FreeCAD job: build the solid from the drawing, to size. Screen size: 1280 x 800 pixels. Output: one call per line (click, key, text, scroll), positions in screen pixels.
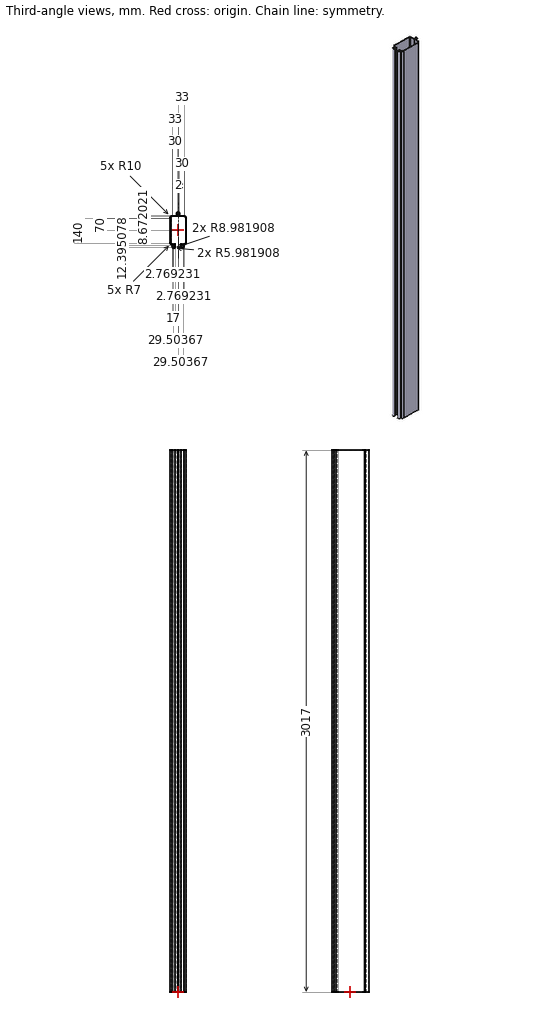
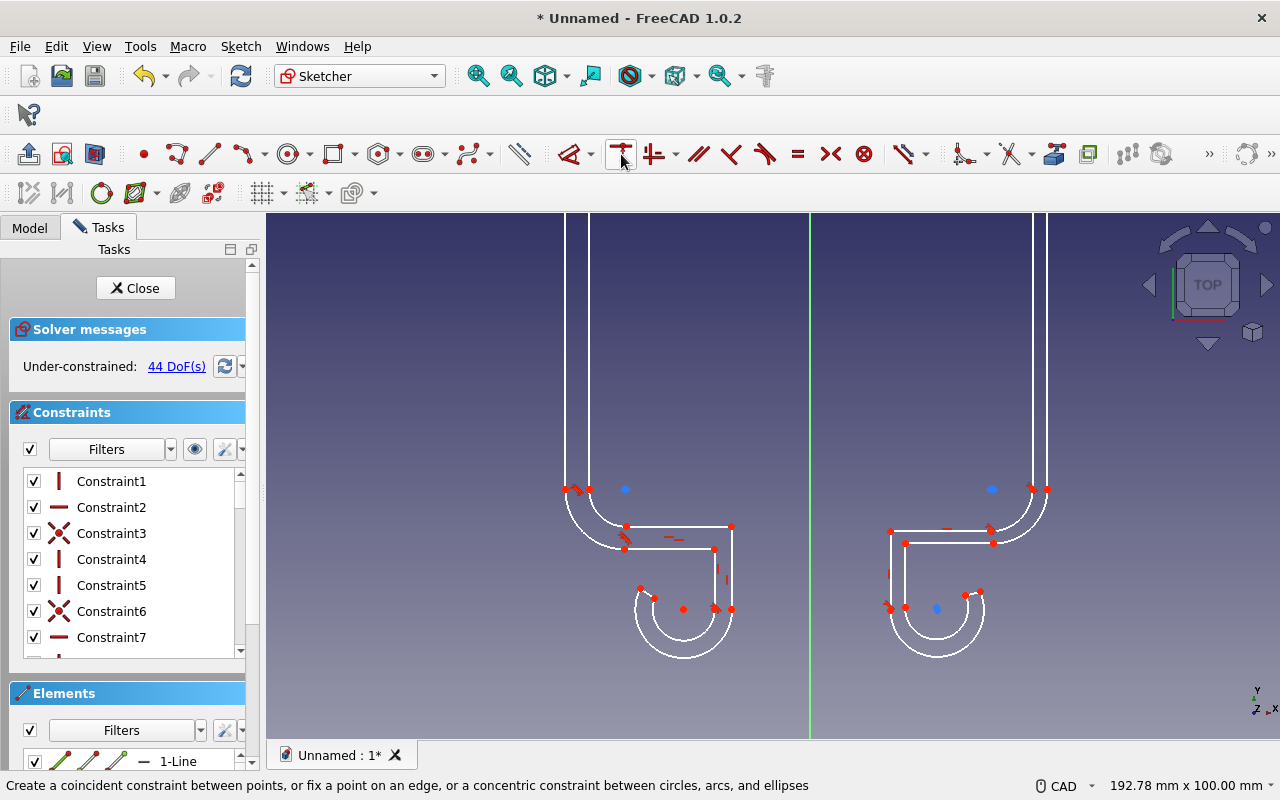
click(572, 517)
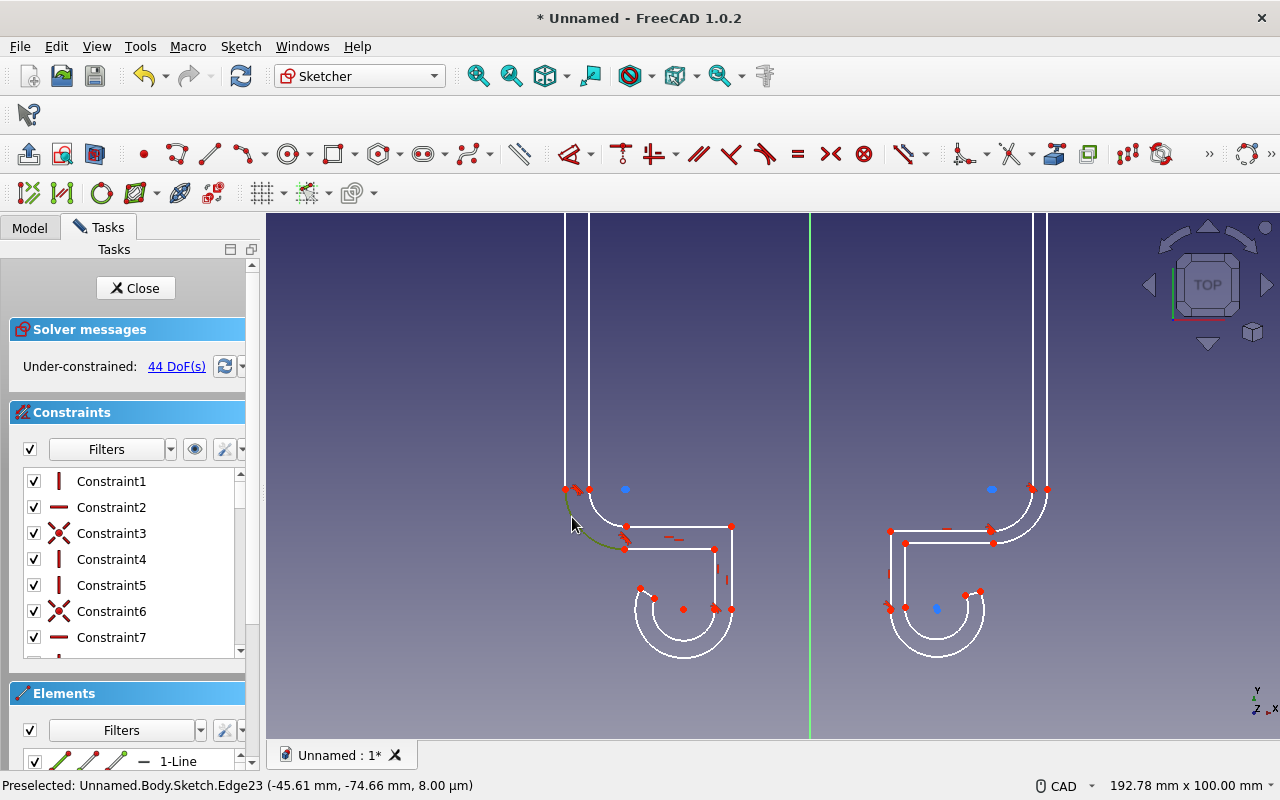
click(593, 507)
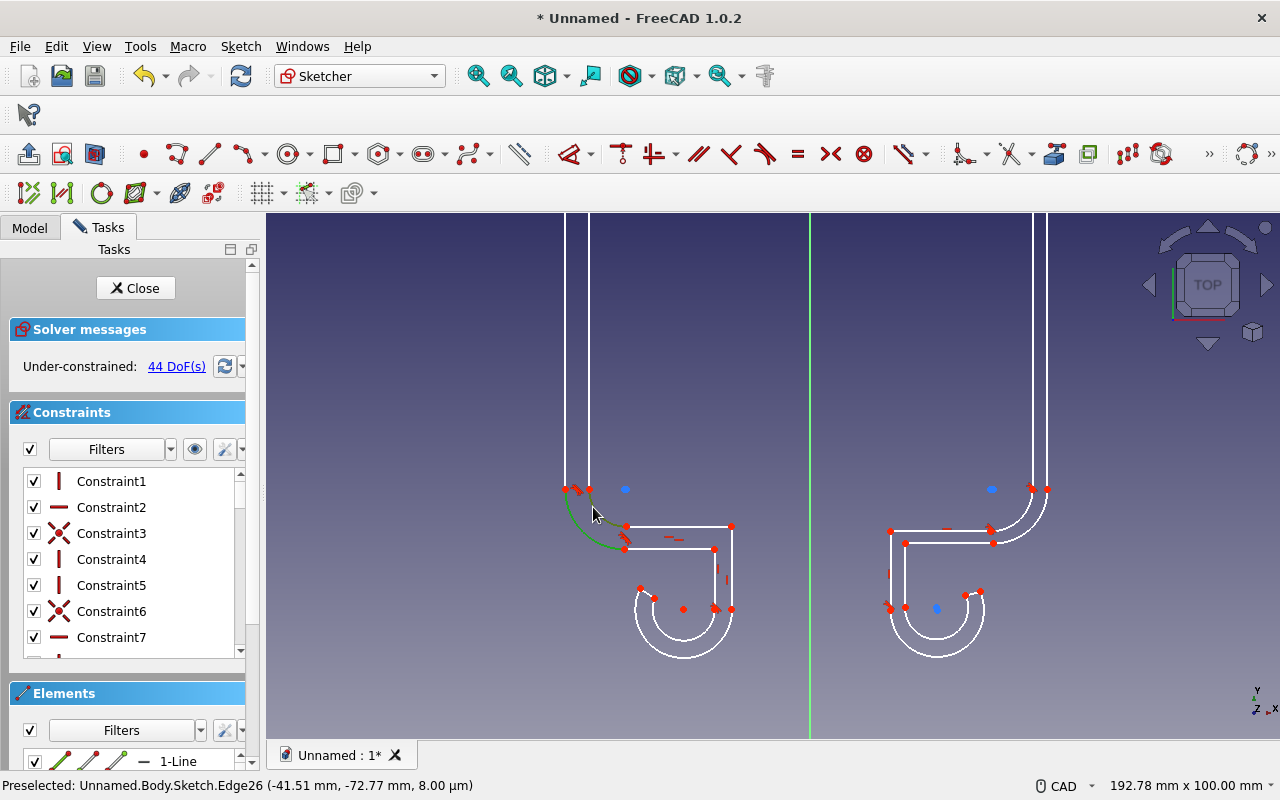
click(621, 154)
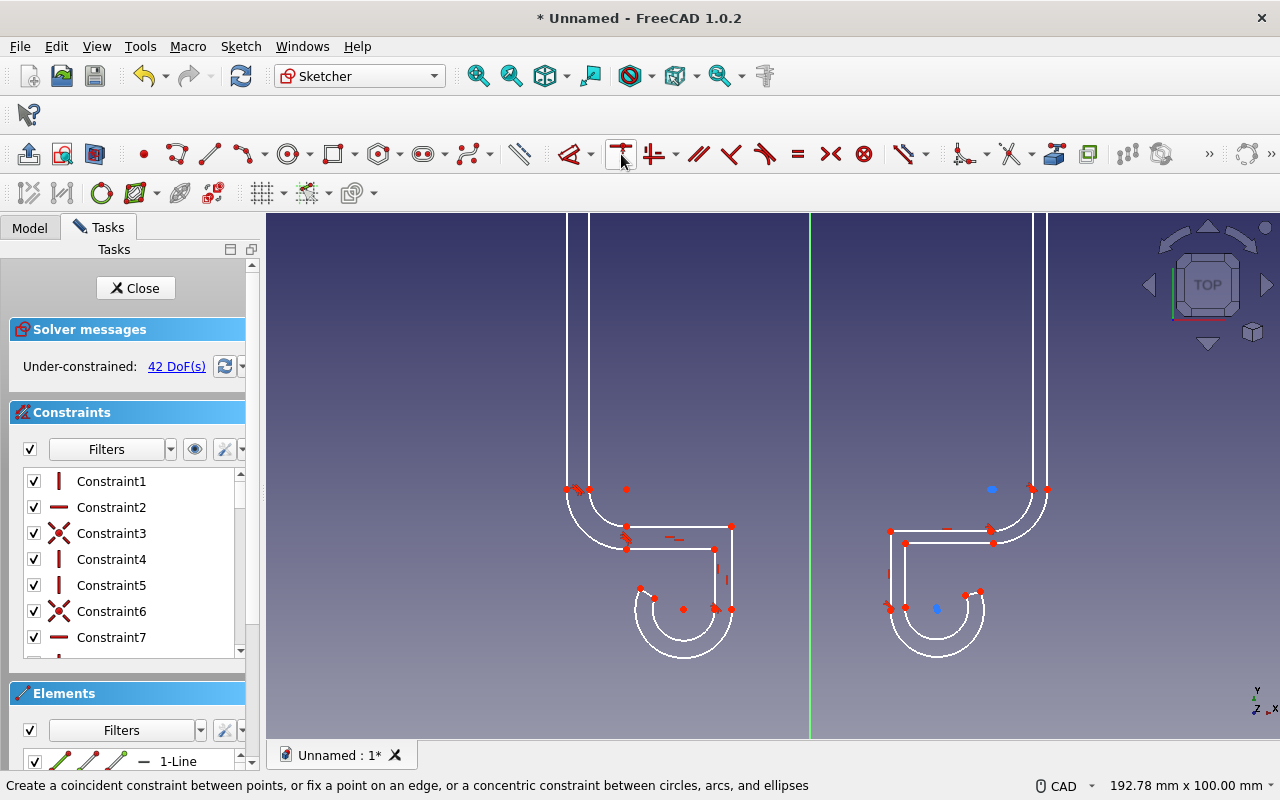
click(915, 651)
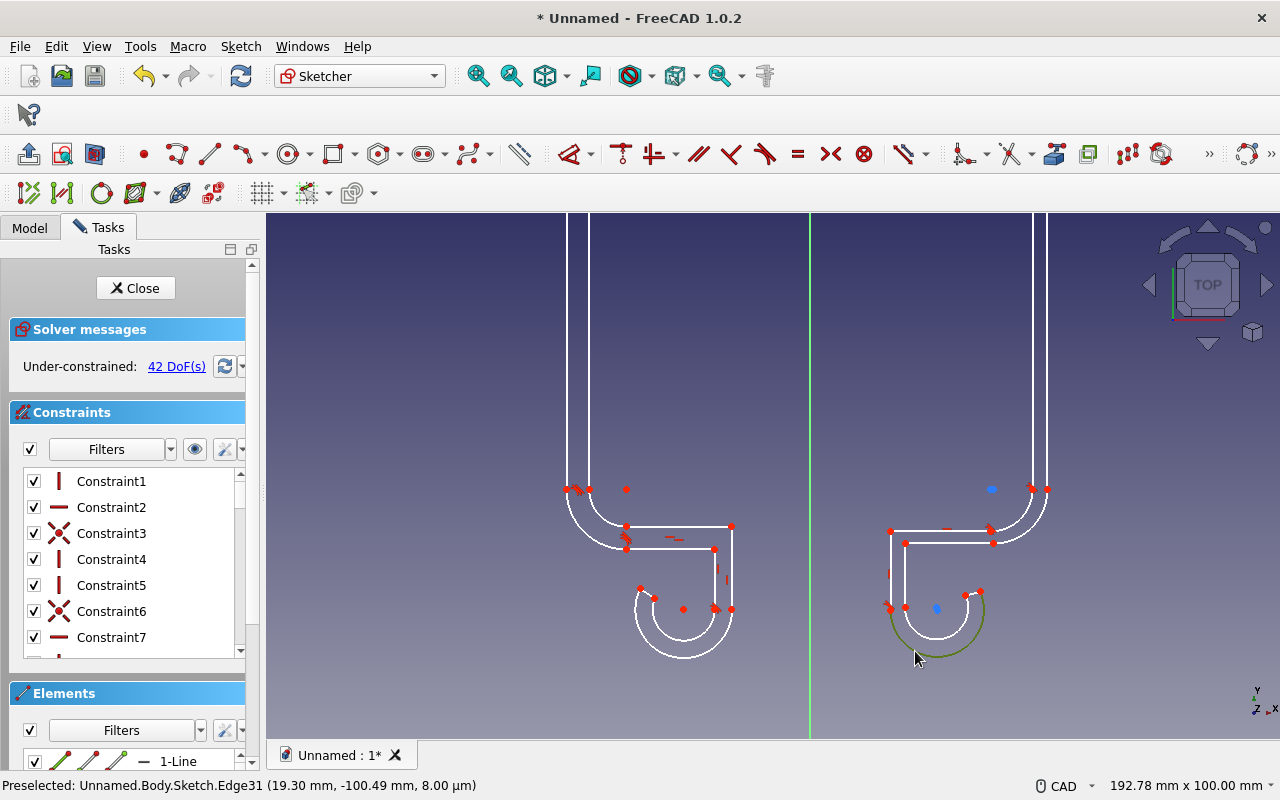
click(921, 635)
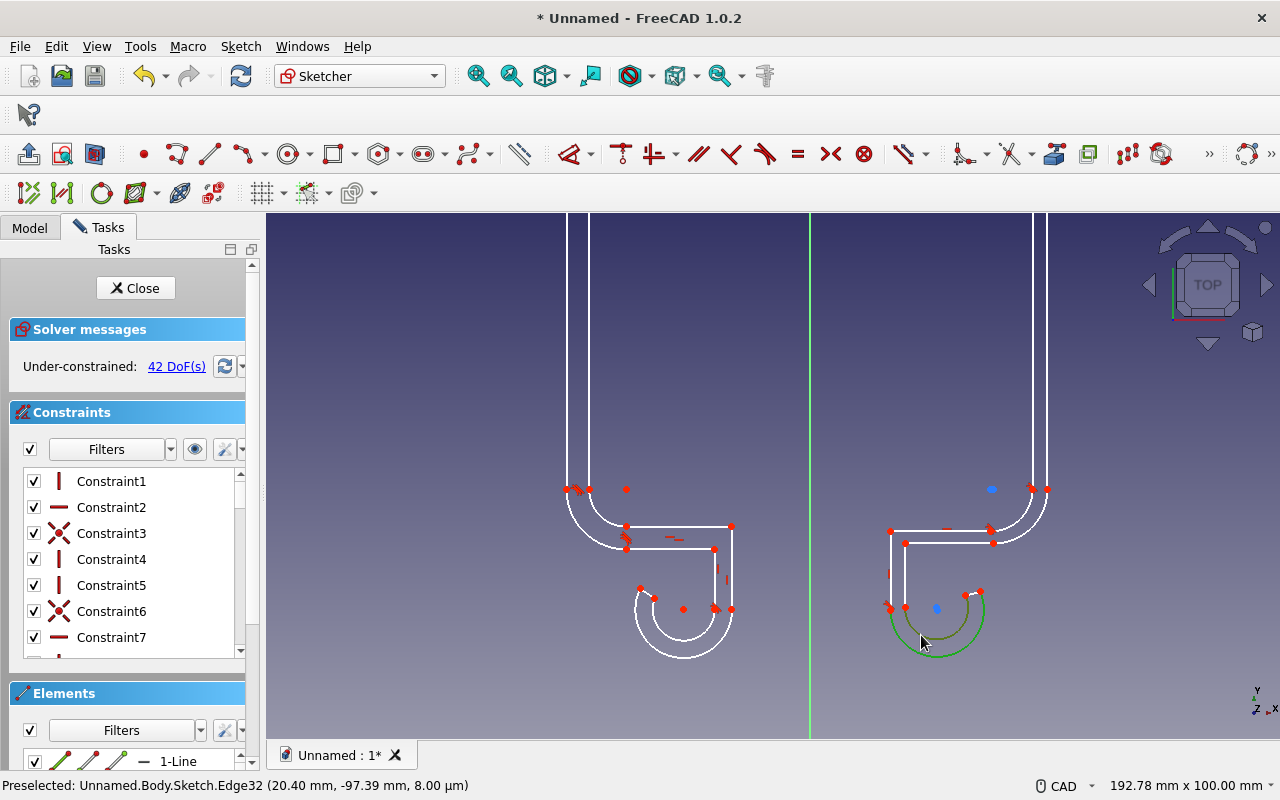
click(621, 154)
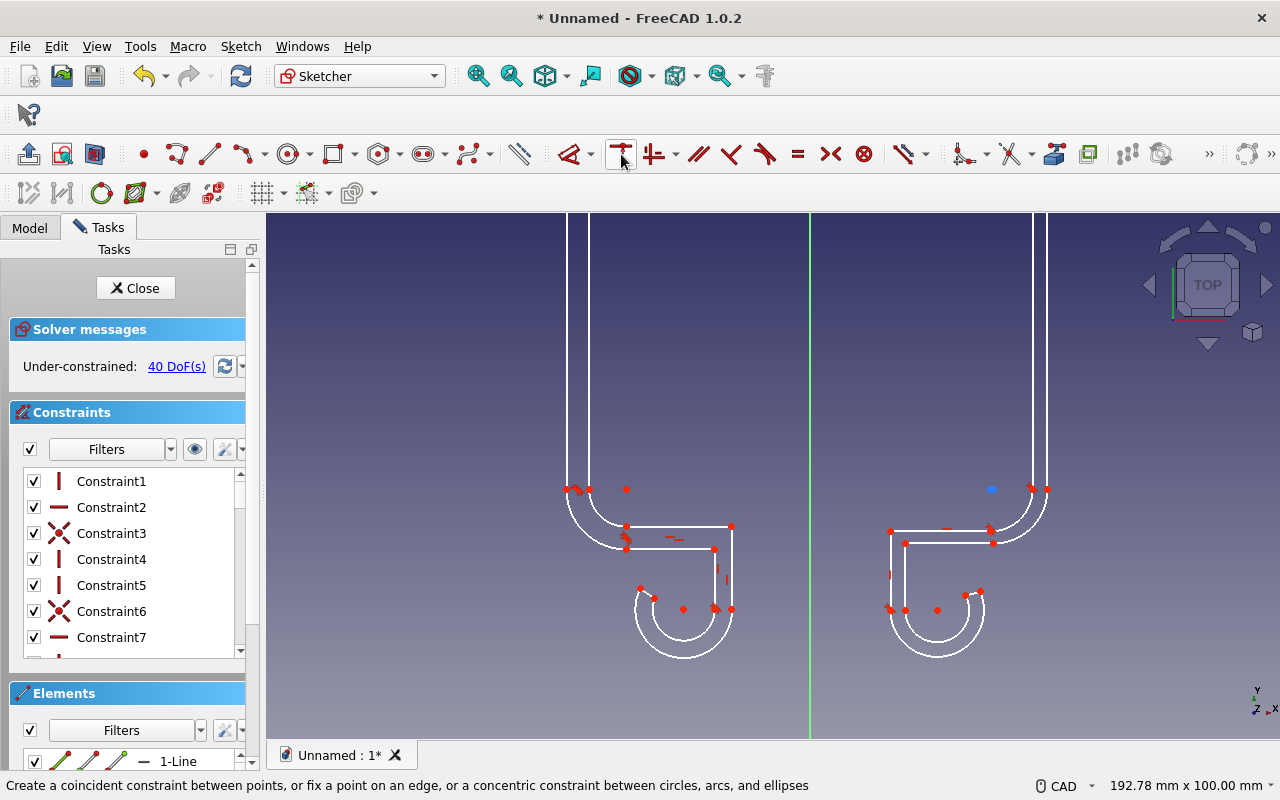
click(1010, 527)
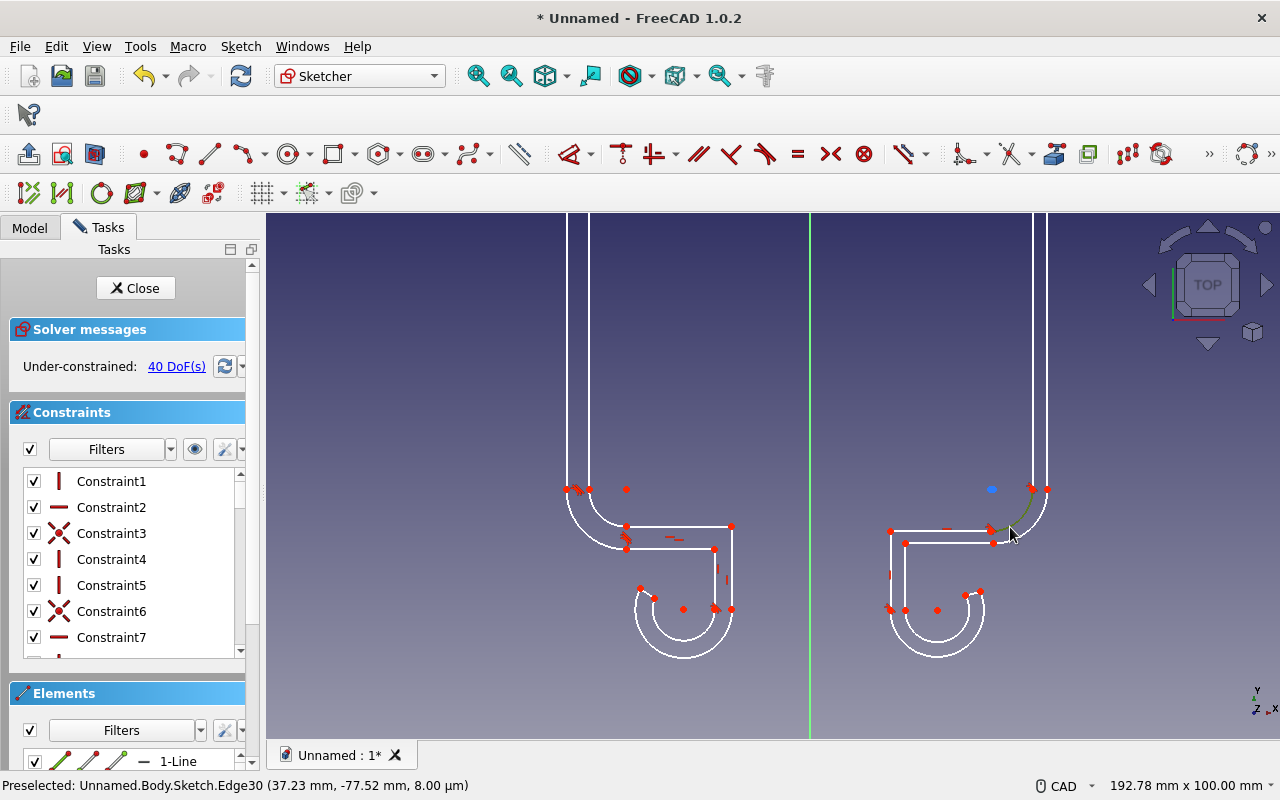
click(1018, 538)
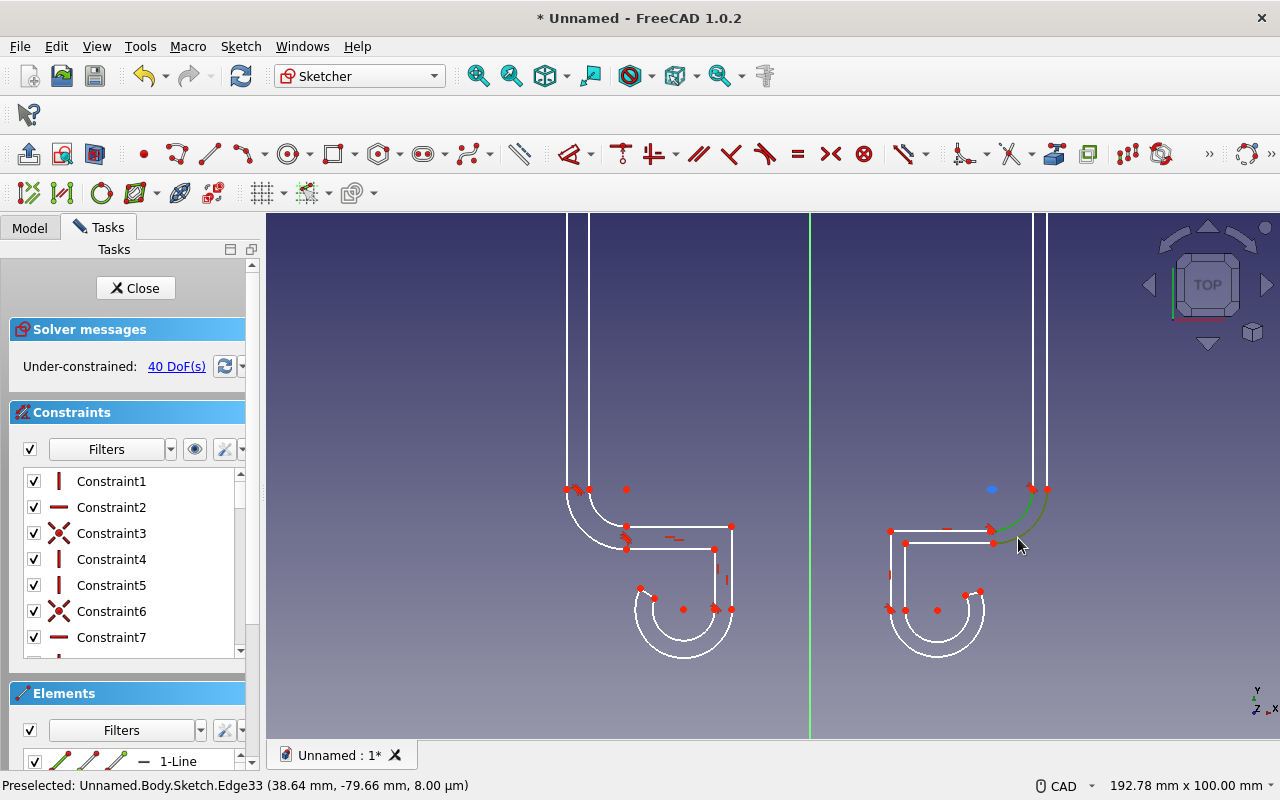
click(621, 154)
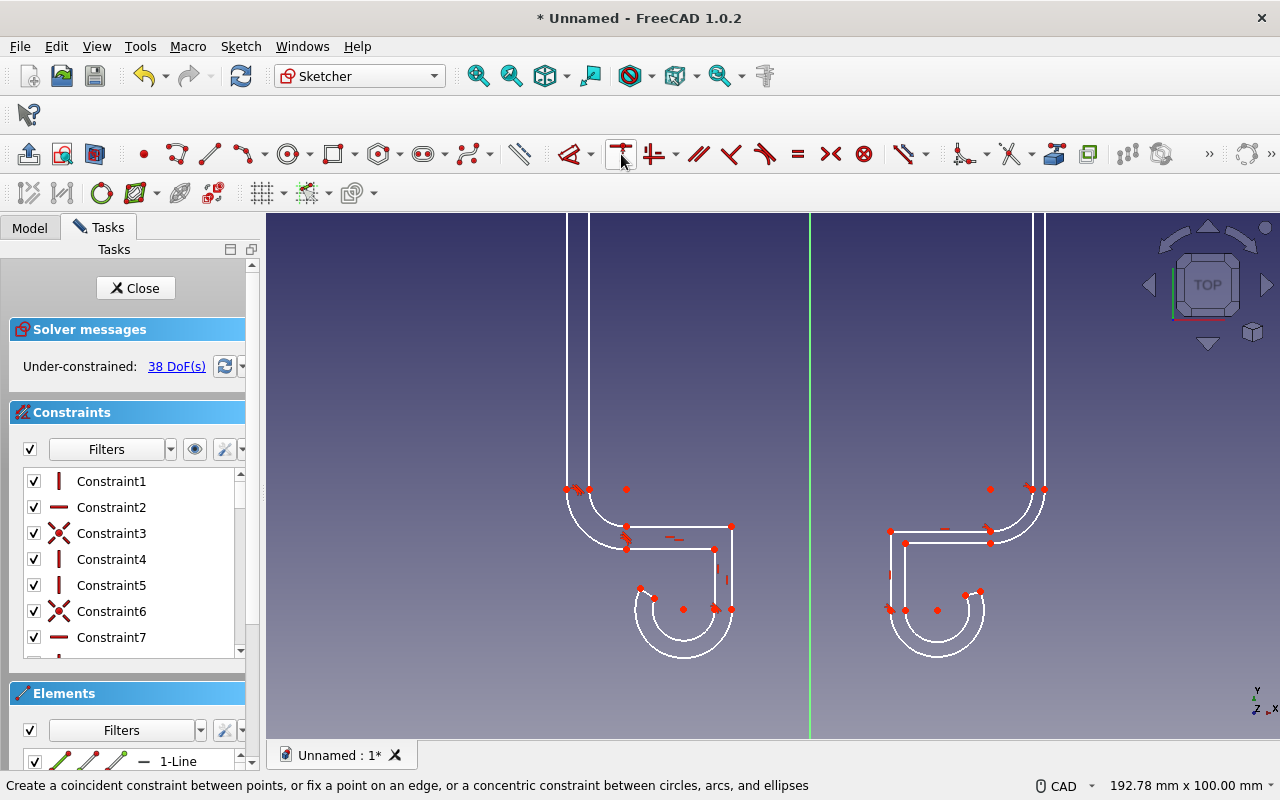
scroll(659, 630, down, 6)